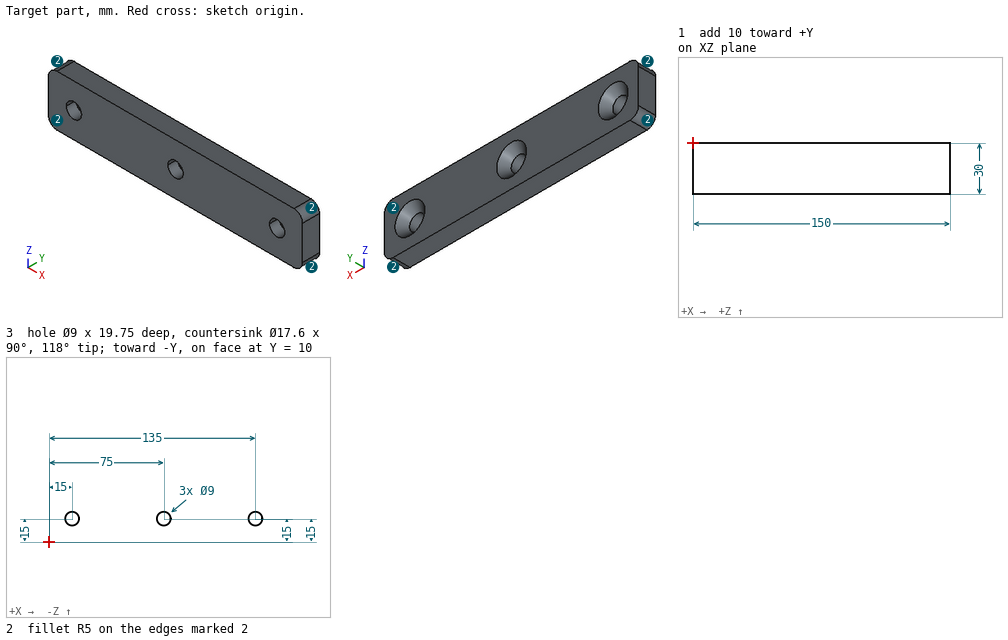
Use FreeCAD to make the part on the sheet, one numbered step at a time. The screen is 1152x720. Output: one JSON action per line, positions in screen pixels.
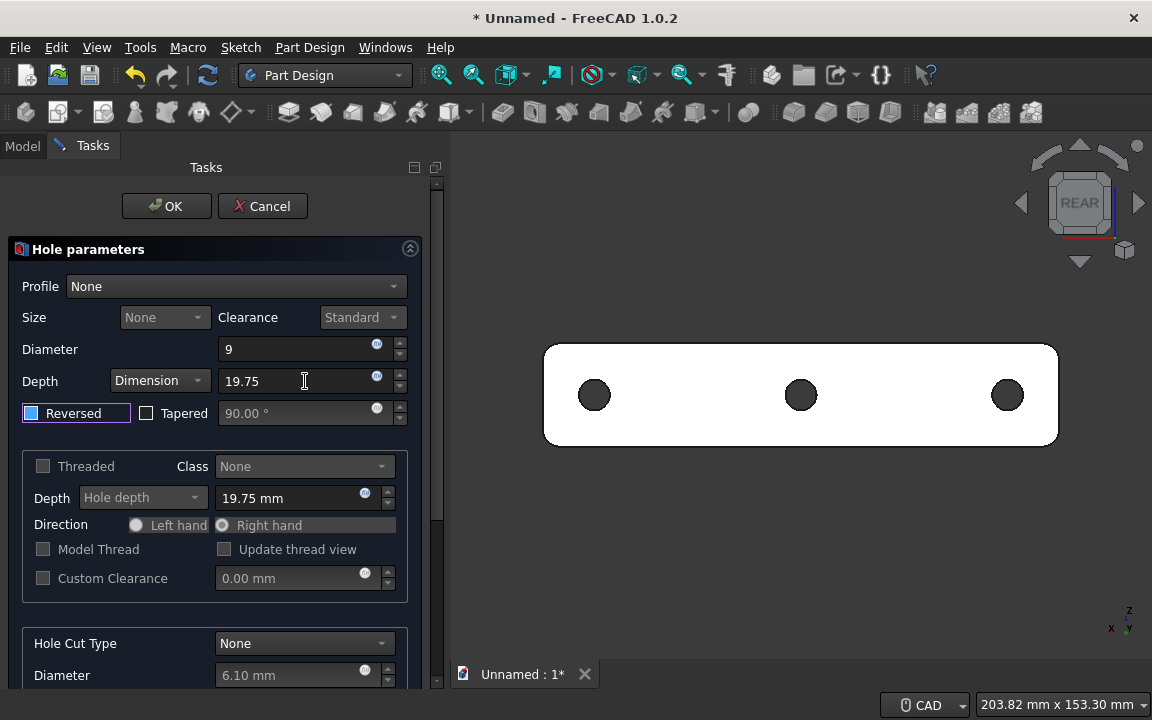
{"action": "left_click", "coordinate": [306, 644]}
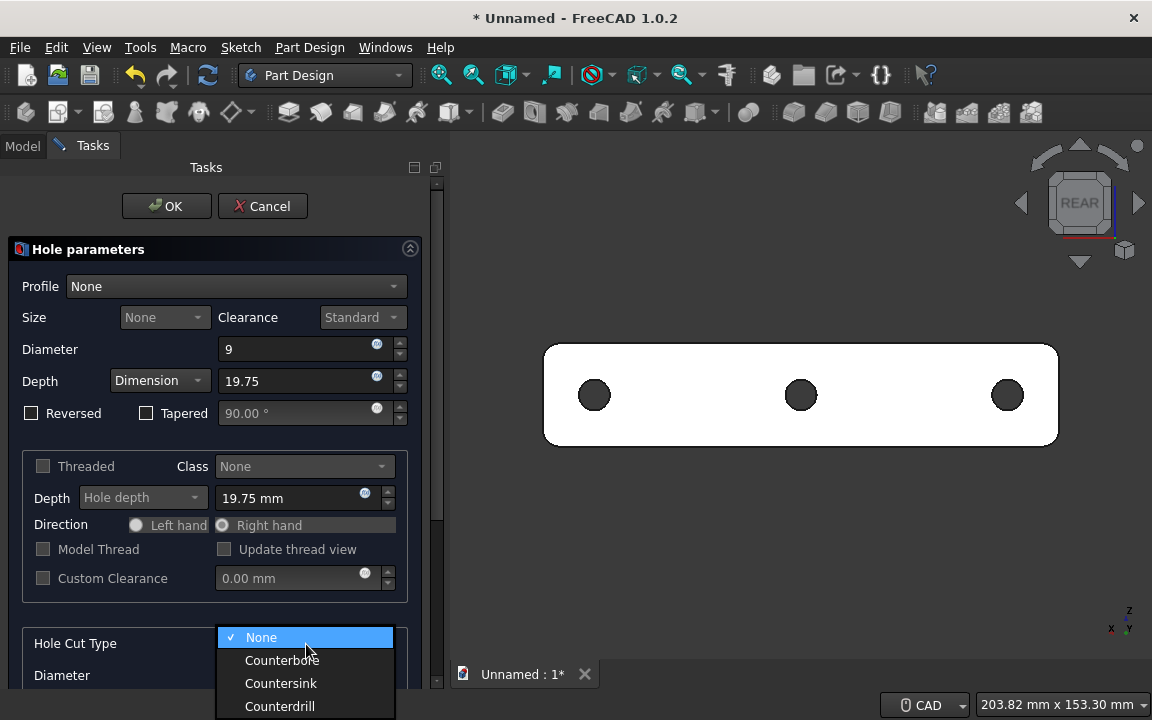
{"action": "left_click", "coordinate": [304, 684]}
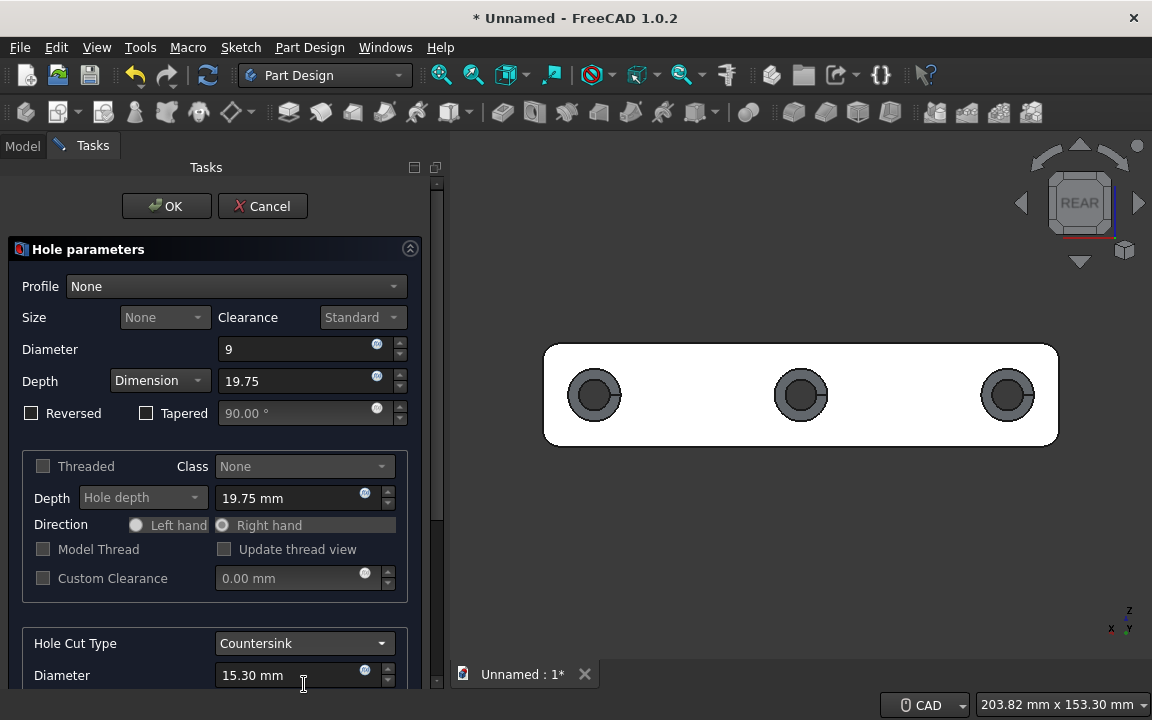
{"action": "triple_click", "coordinate": [298, 675]}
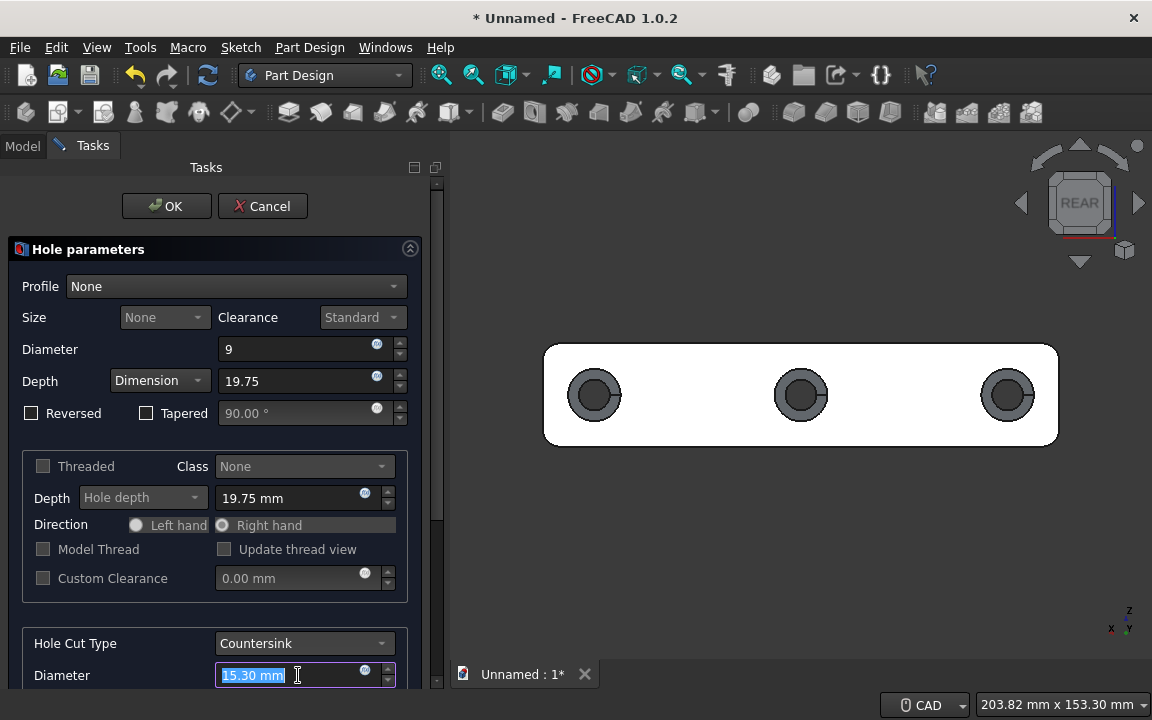
{"action": "type", "text": "17.6"}
{"action": "key", "text": "Tab"}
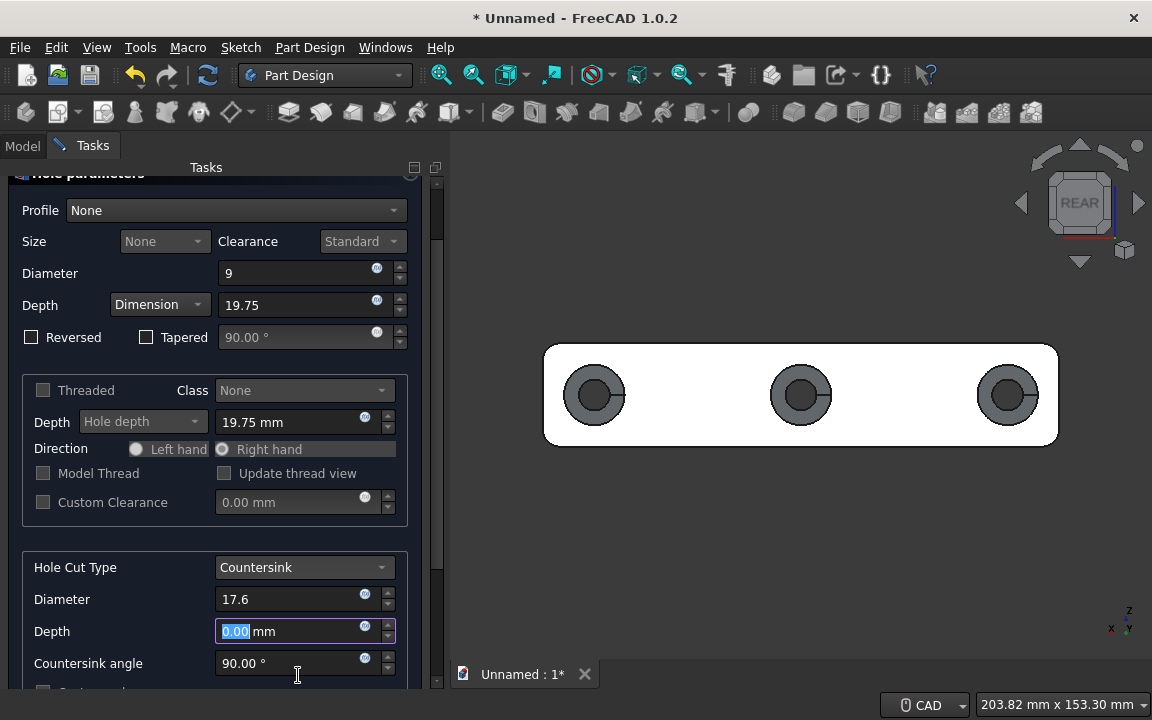
{"action": "scroll", "coordinate": [437, 432], "scroll_direction": "up", "scroll_amount": 3}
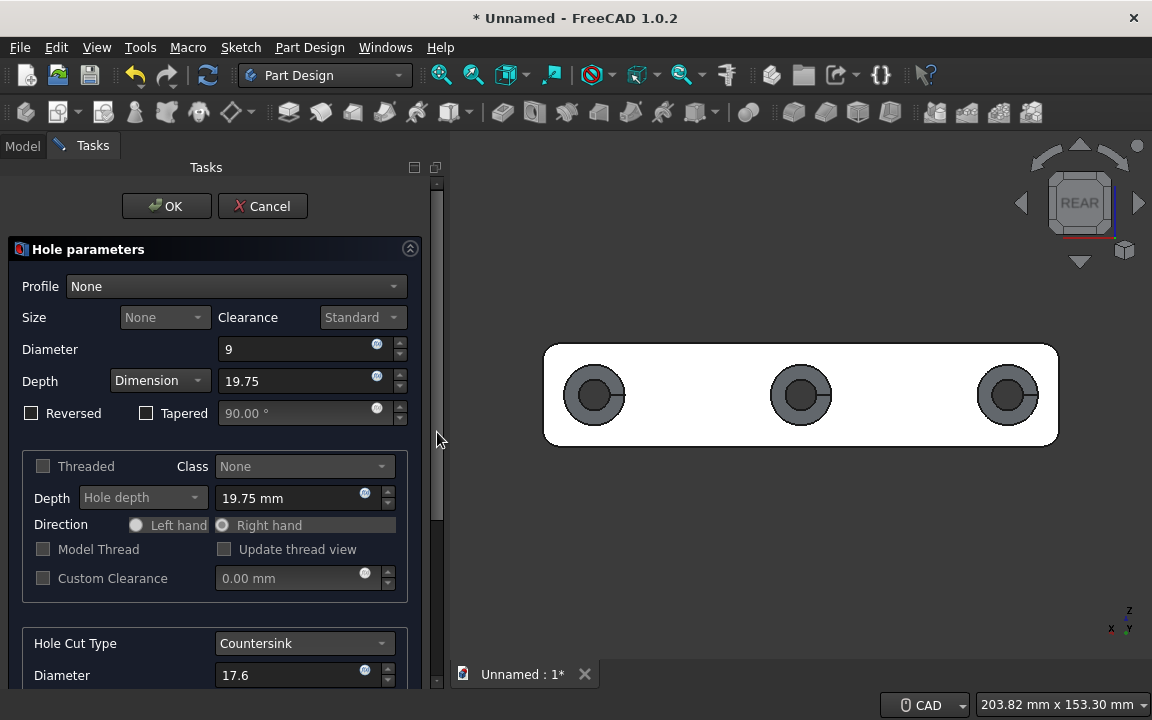
{"action": "left_click", "coordinate": [167, 206]}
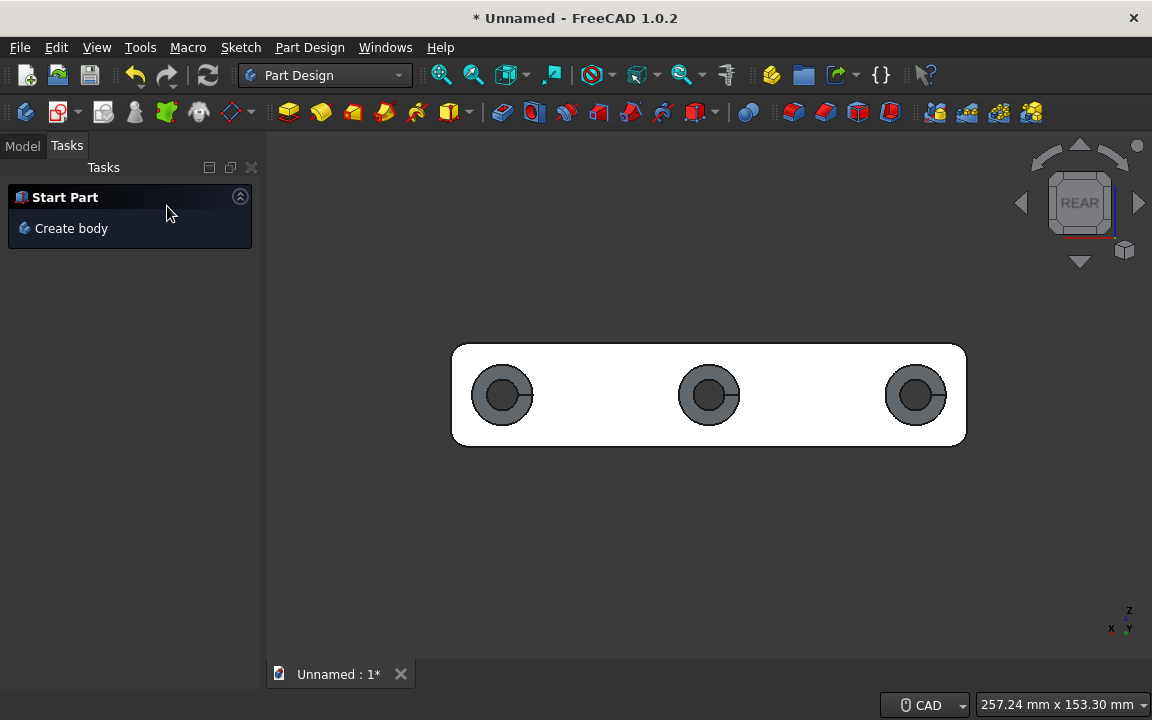
{"action": "key", "text": "0"}